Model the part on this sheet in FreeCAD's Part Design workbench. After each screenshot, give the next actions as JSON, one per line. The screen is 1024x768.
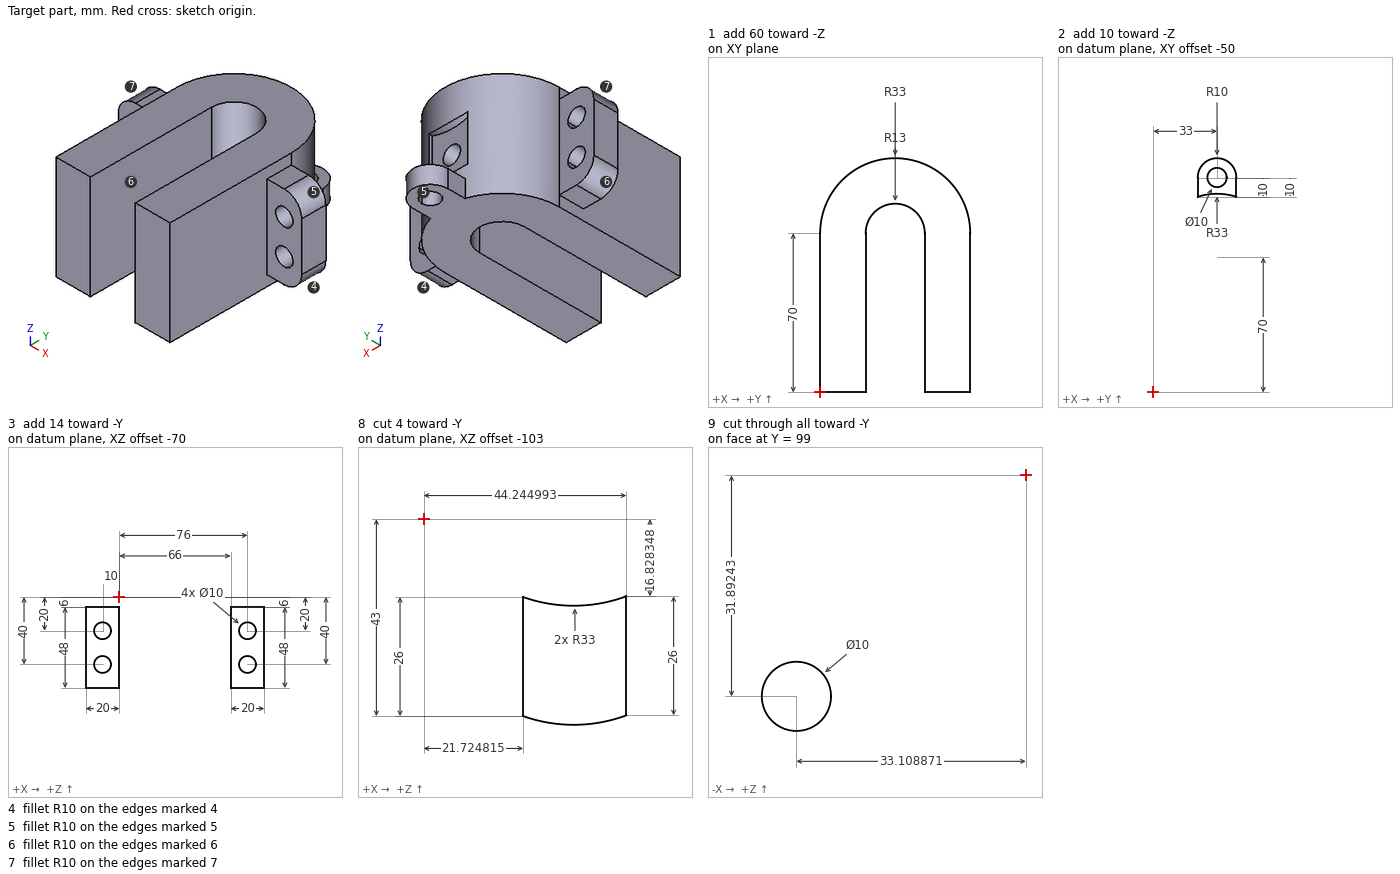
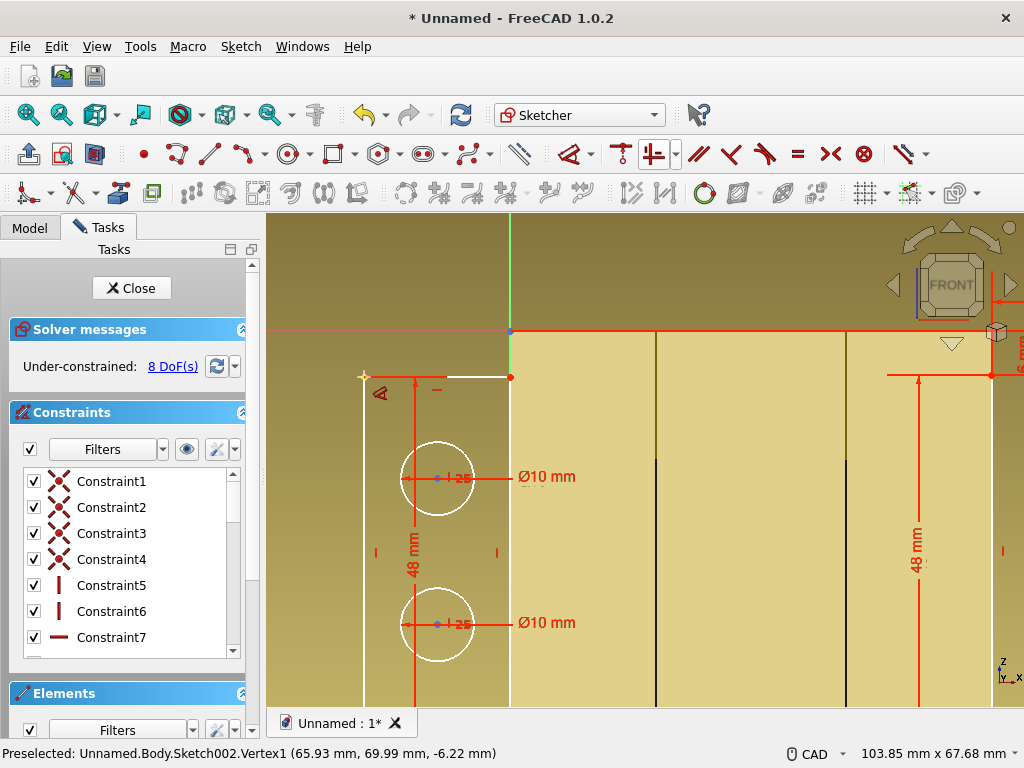
{"action": "left_click", "coordinate": [364, 377]}
{"action": "left_click", "coordinate": [330, 354]}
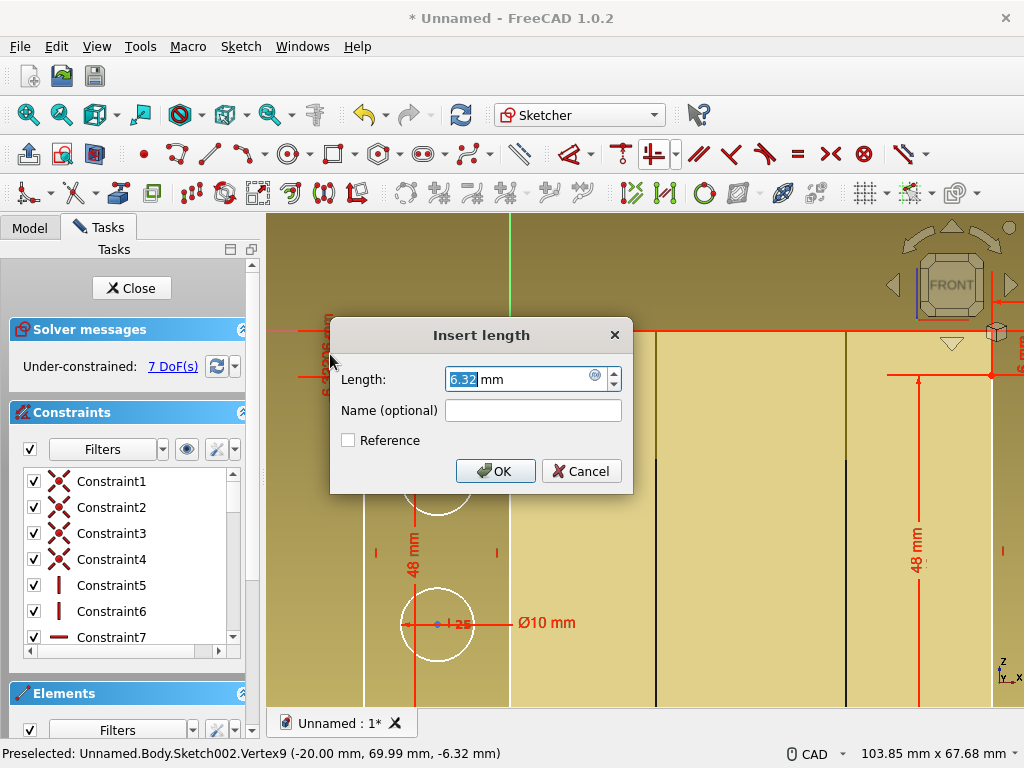
{"action": "type", "text": "6"}
{"action": "key", "text": "Return"}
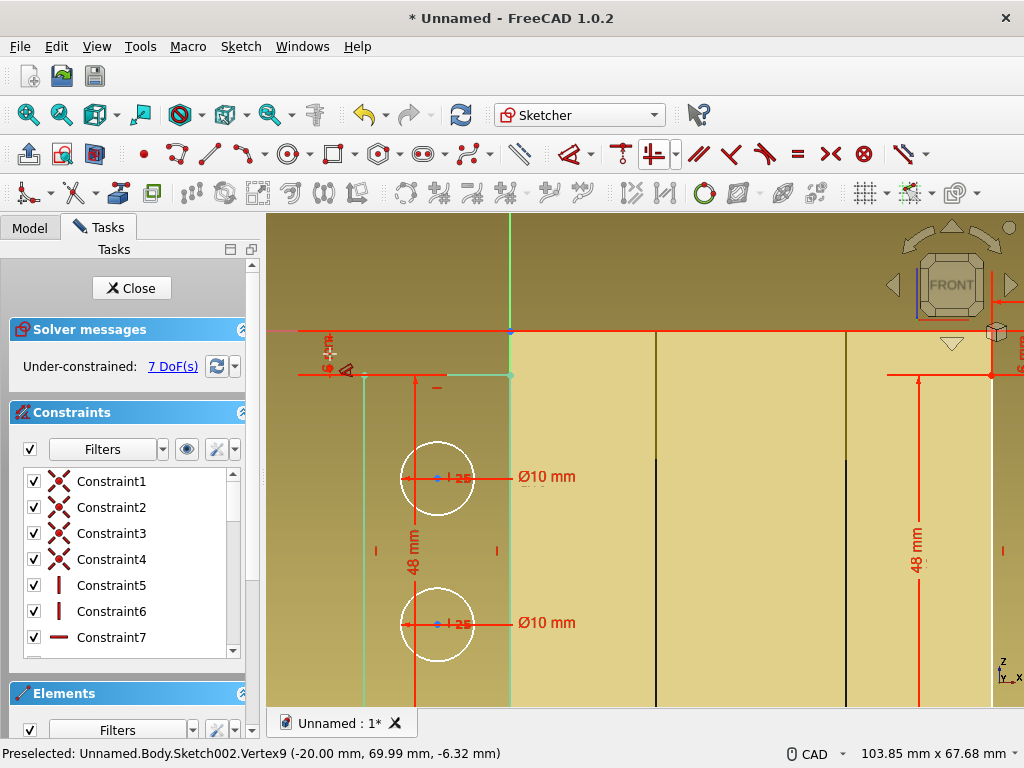
{"action": "scroll", "coordinate": [364, 377], "scroll_direction": "down", "scroll_amount": 3}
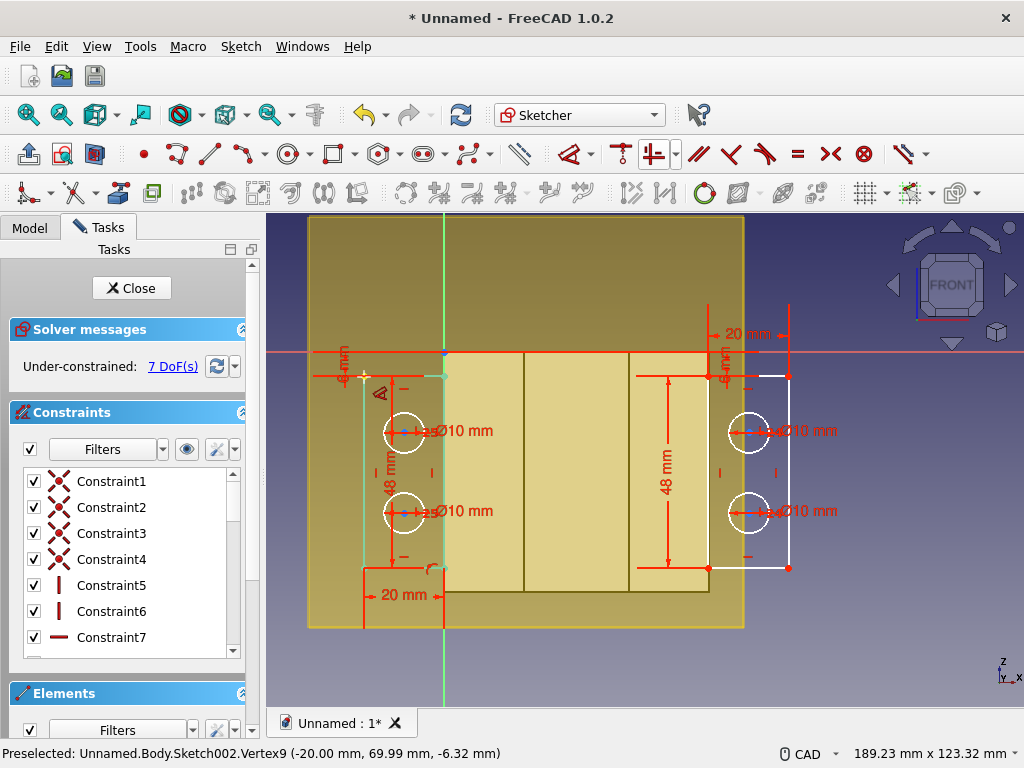
{"action": "left_click", "coordinate": [749, 433]}
{"action": "left_click", "coordinate": [597, 318]}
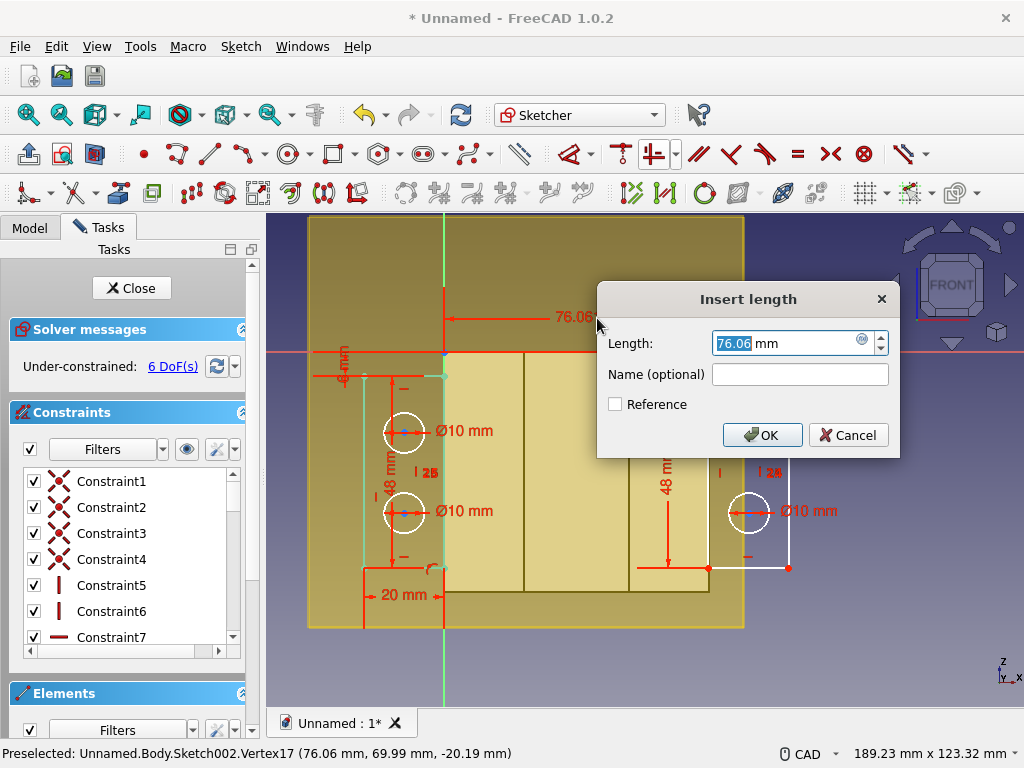
{"action": "type", "text": "76"}
{"action": "key", "text": "Return"}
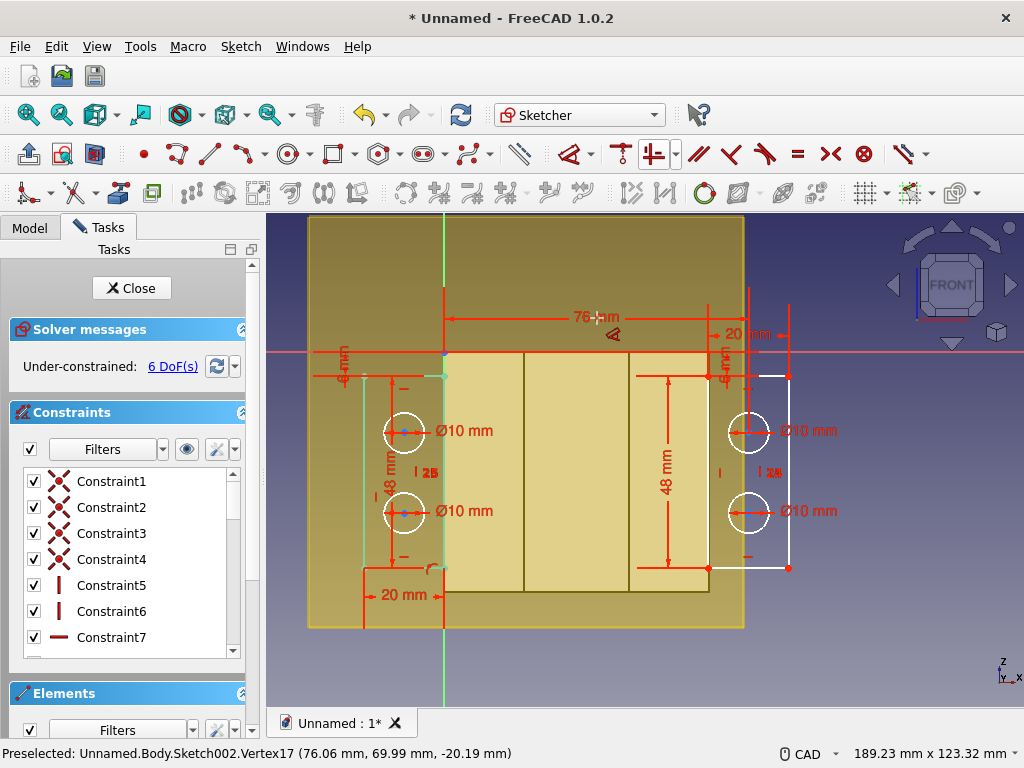
{"action": "left_click", "coordinate": [749, 433]}
{"action": "left_click", "coordinate": [410, 392]}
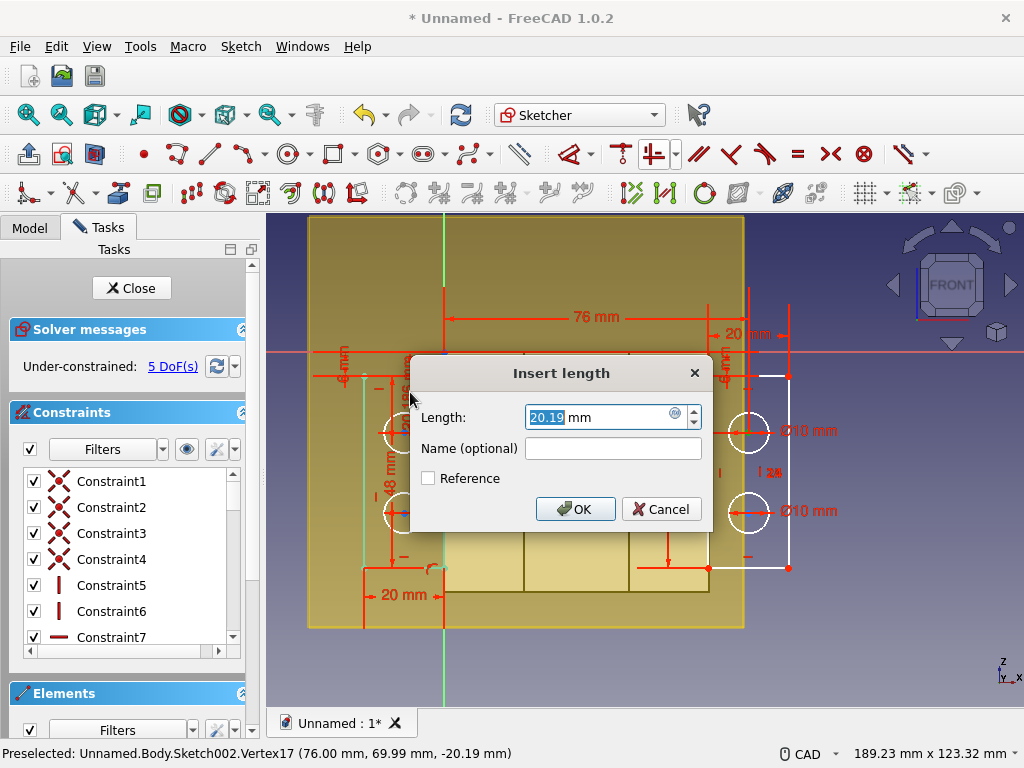
{"action": "type", "text": "20"}
{"action": "key", "text": "Return"}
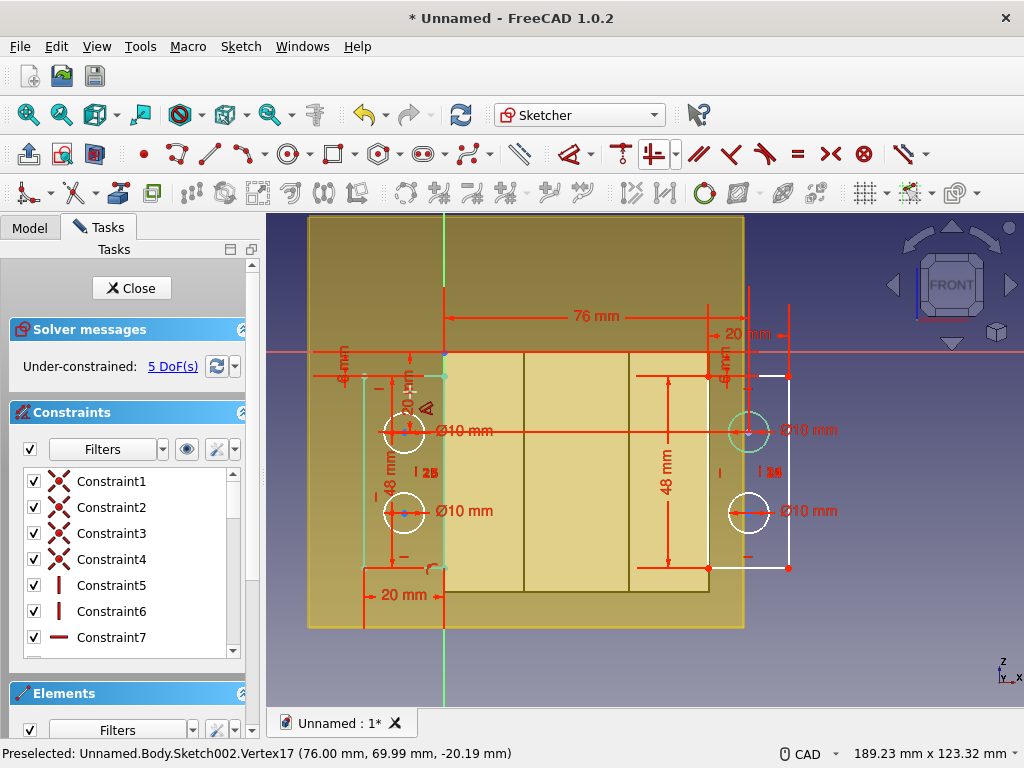
{"action": "left_click", "coordinate": [749, 513]}
{"action": "left_click", "coordinate": [410, 433]}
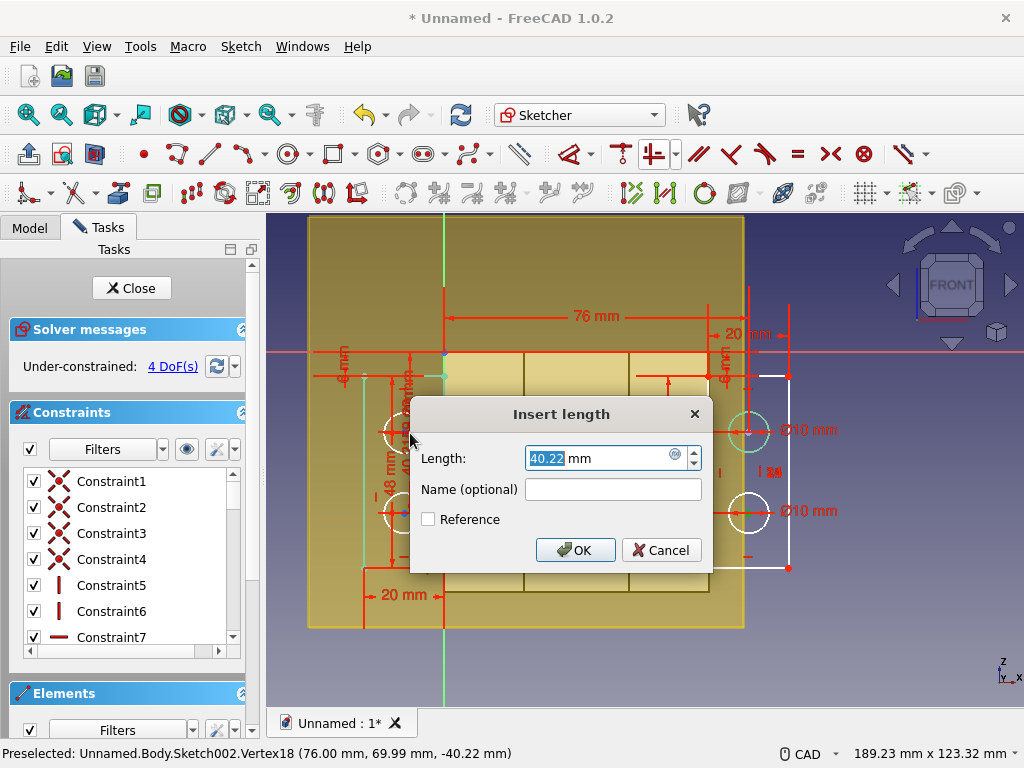
{"action": "type", "text": "40"}
{"action": "key", "text": "Return"}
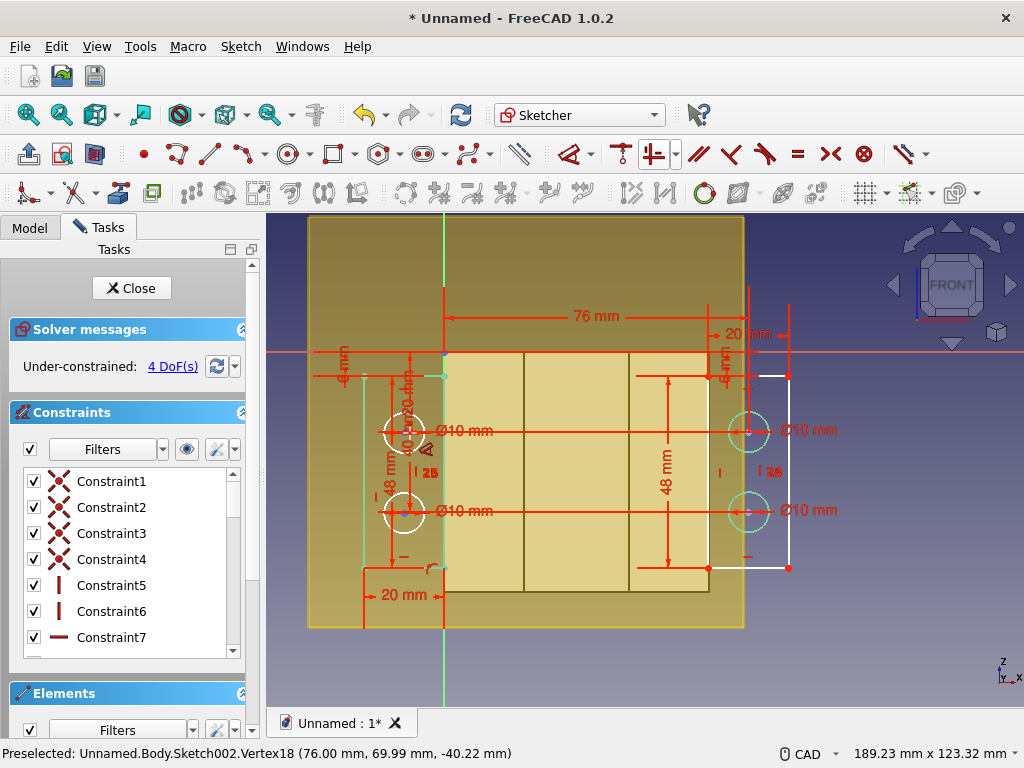
{"action": "left_click", "coordinate": [404, 433]}
{"action": "left_click", "coordinate": [424, 318]}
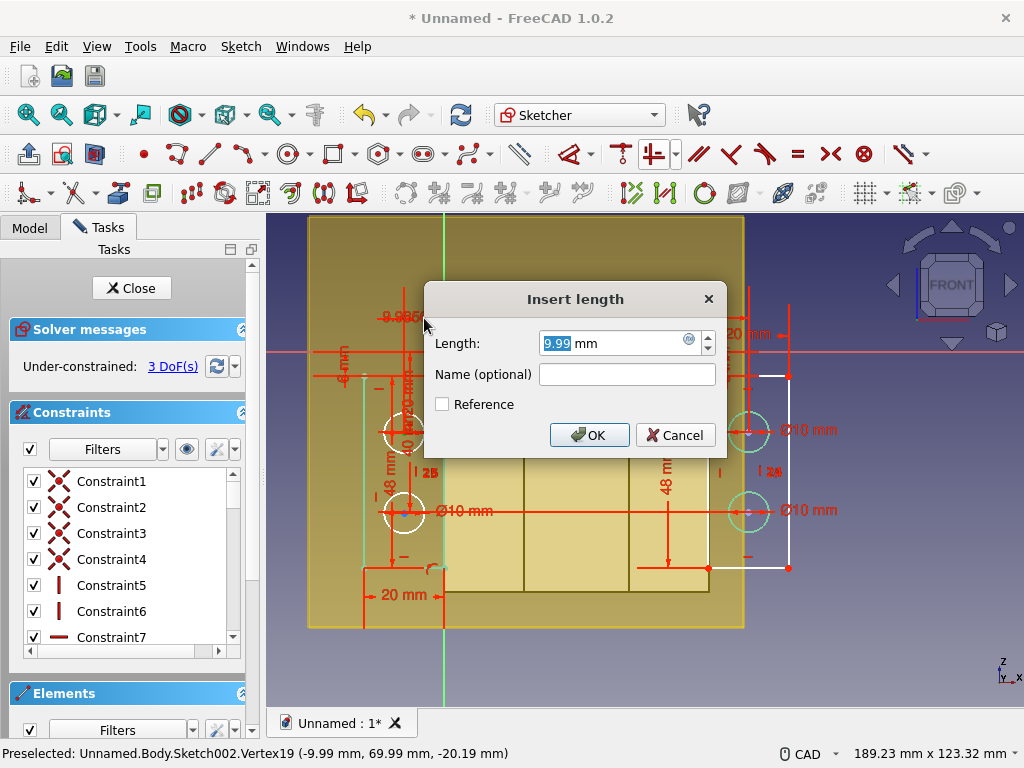
{"action": "type", "text": "10"}
{"action": "key", "text": "Return"}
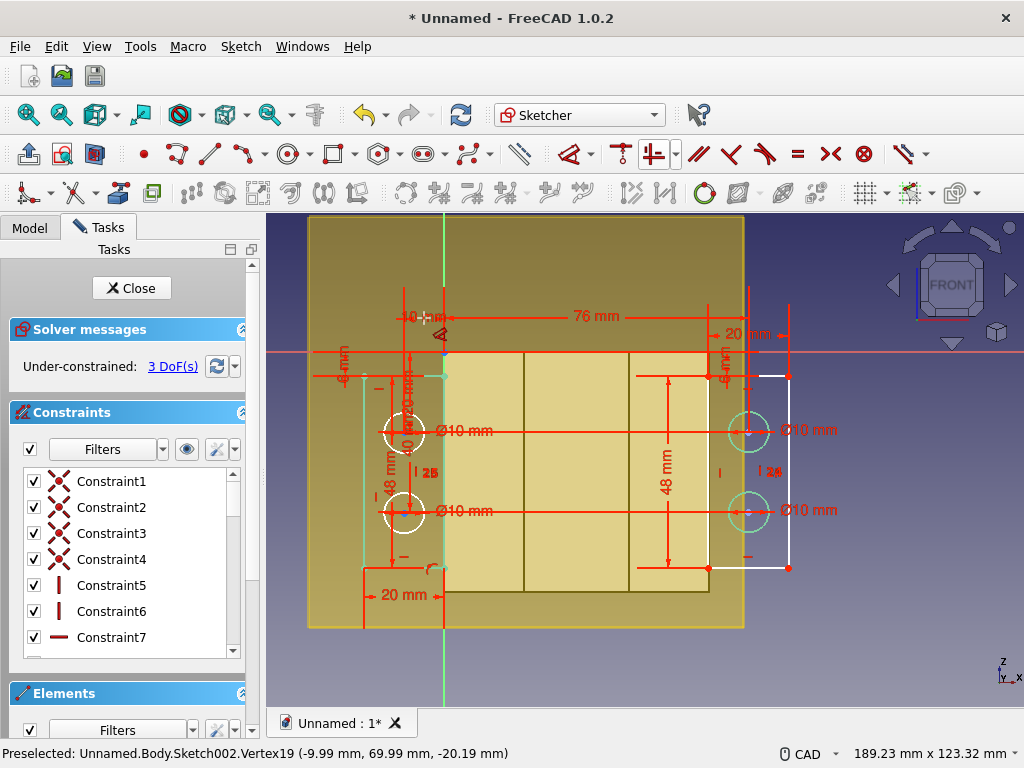
{"action": "left_click", "coordinate": [404, 433]}
{"action": "left_click", "coordinate": [502, 392]}